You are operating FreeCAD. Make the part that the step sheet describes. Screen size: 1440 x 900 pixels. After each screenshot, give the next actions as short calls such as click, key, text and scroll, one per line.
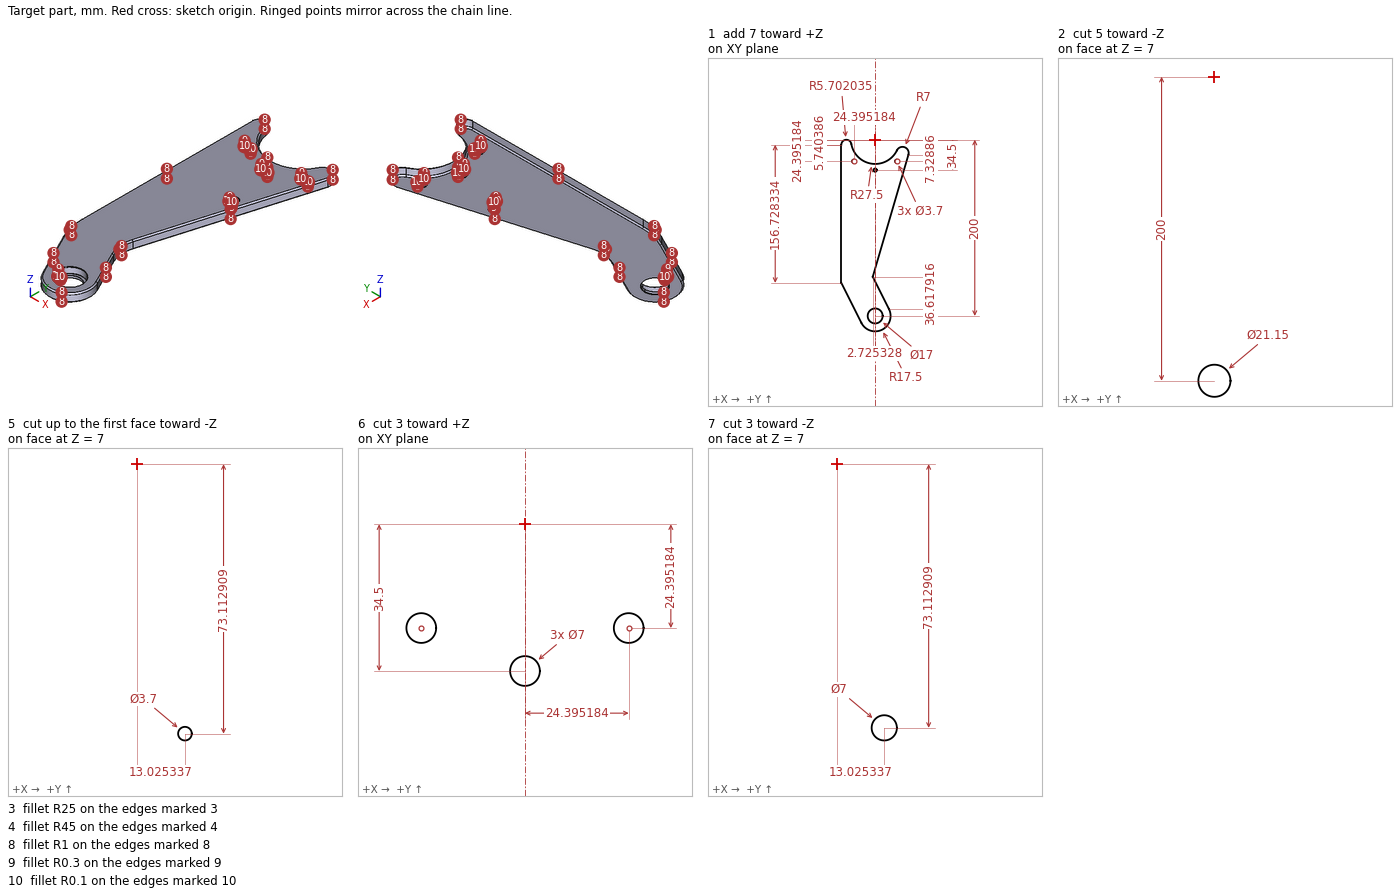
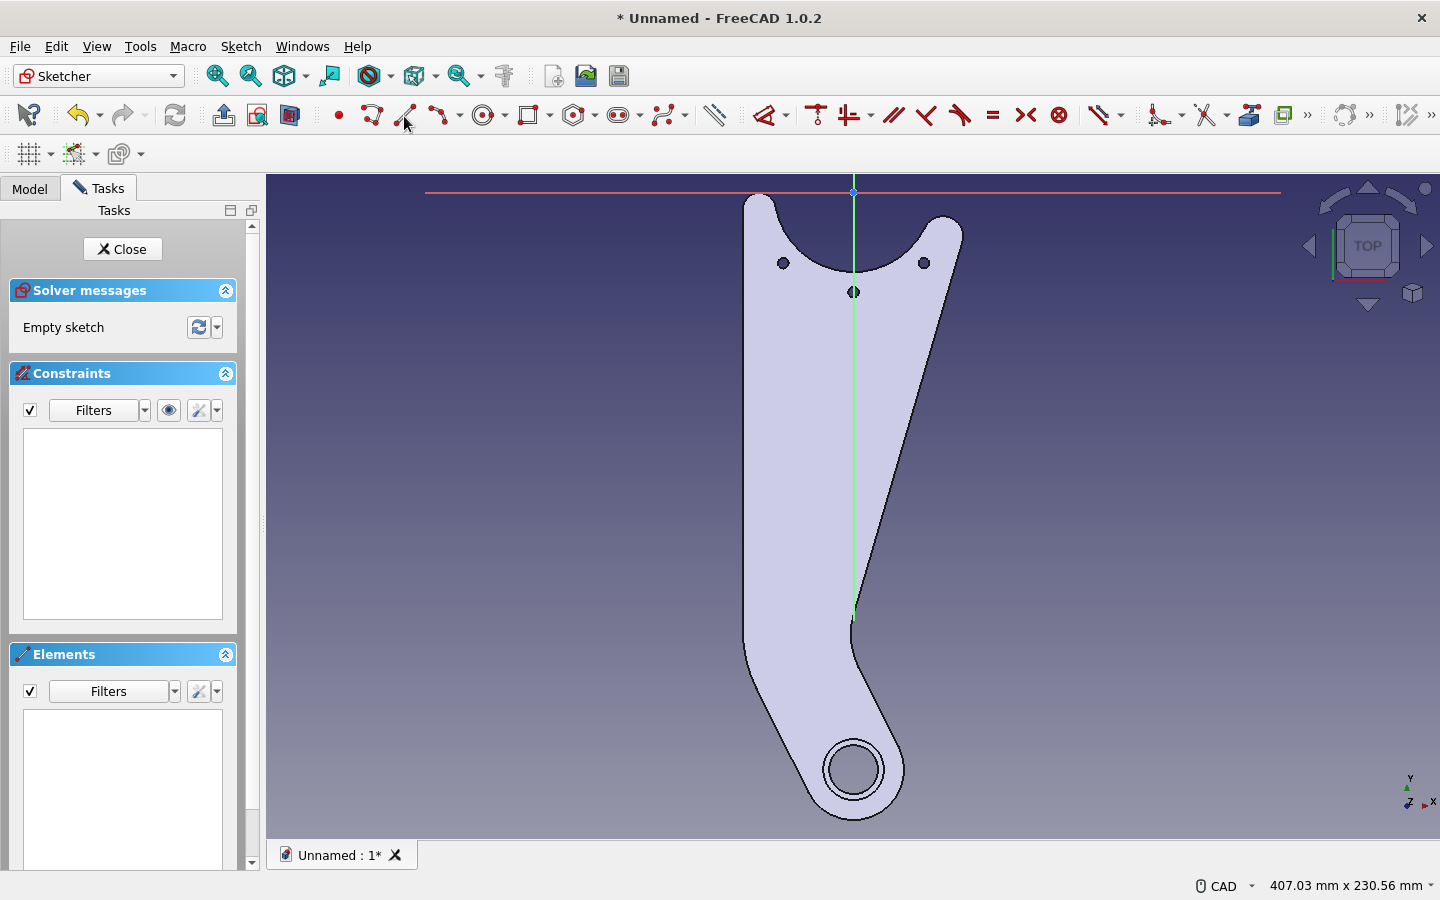
scroll(897, 398, up, 15)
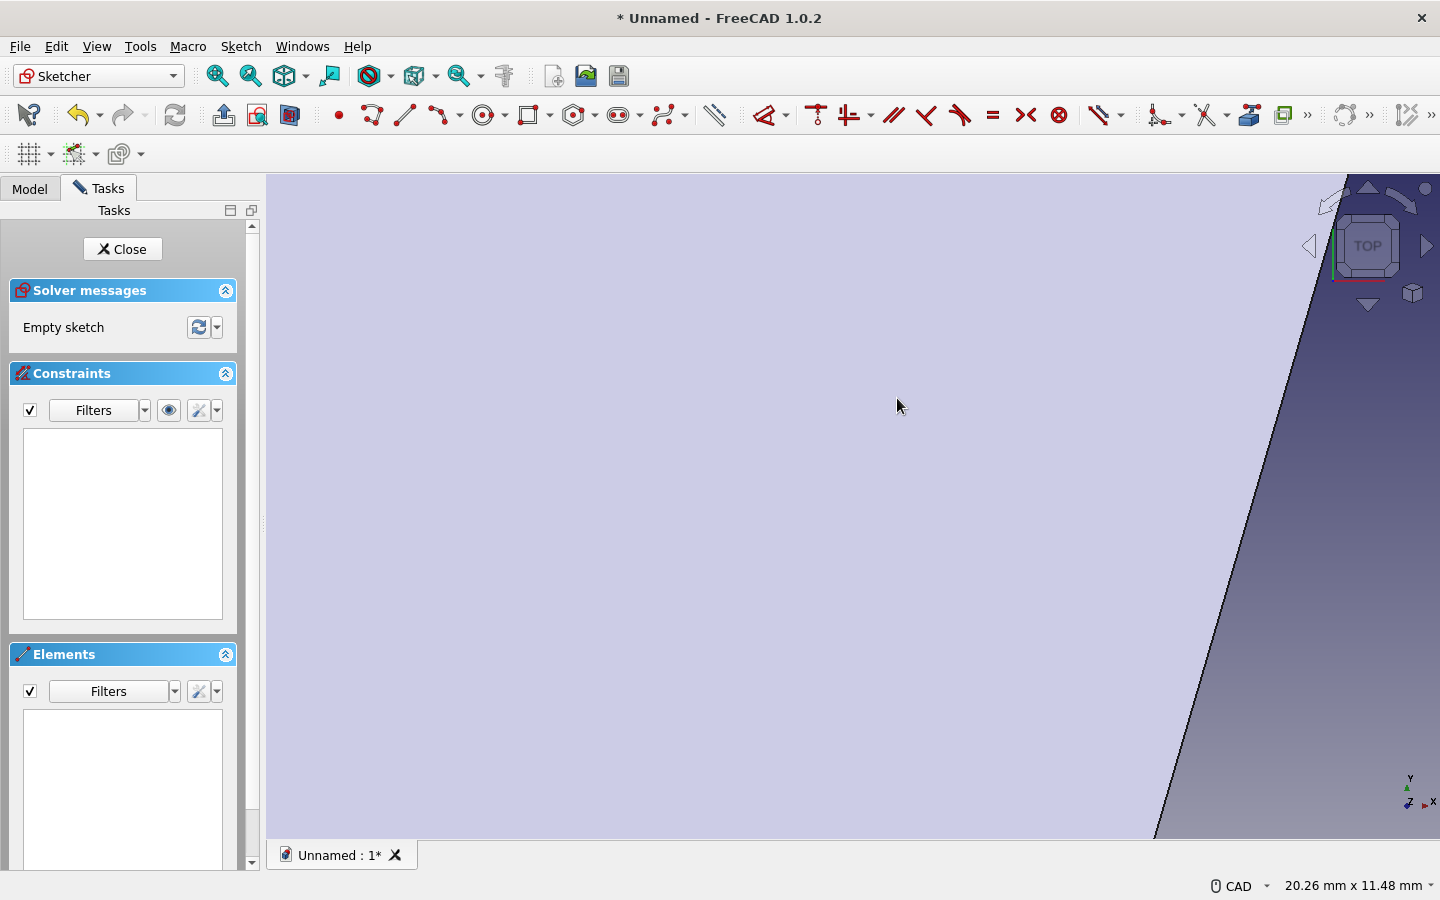
scroll(750, 504, up, 3)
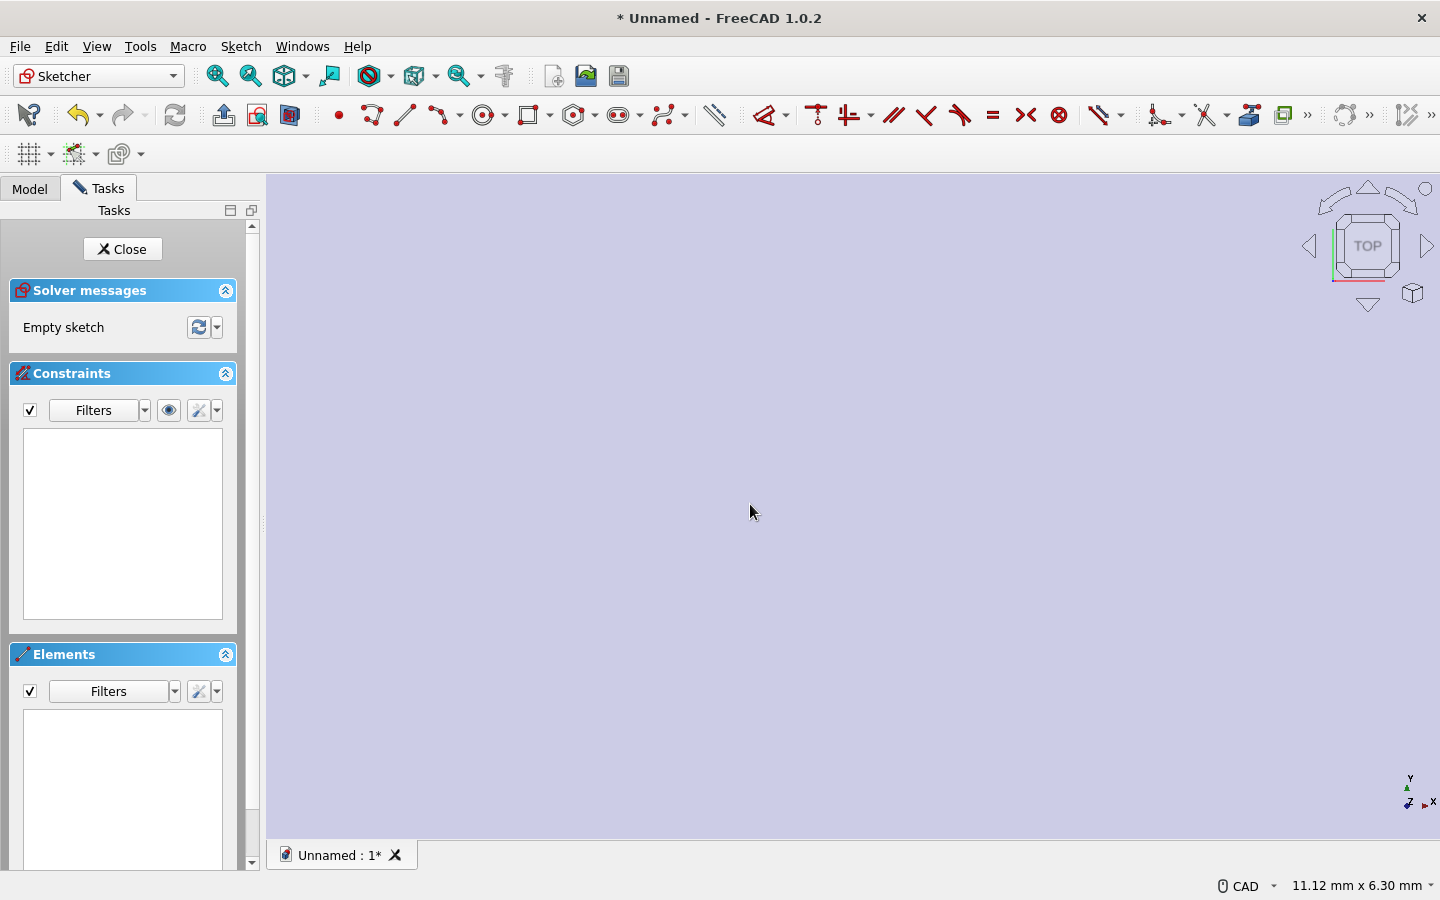
click(482, 116)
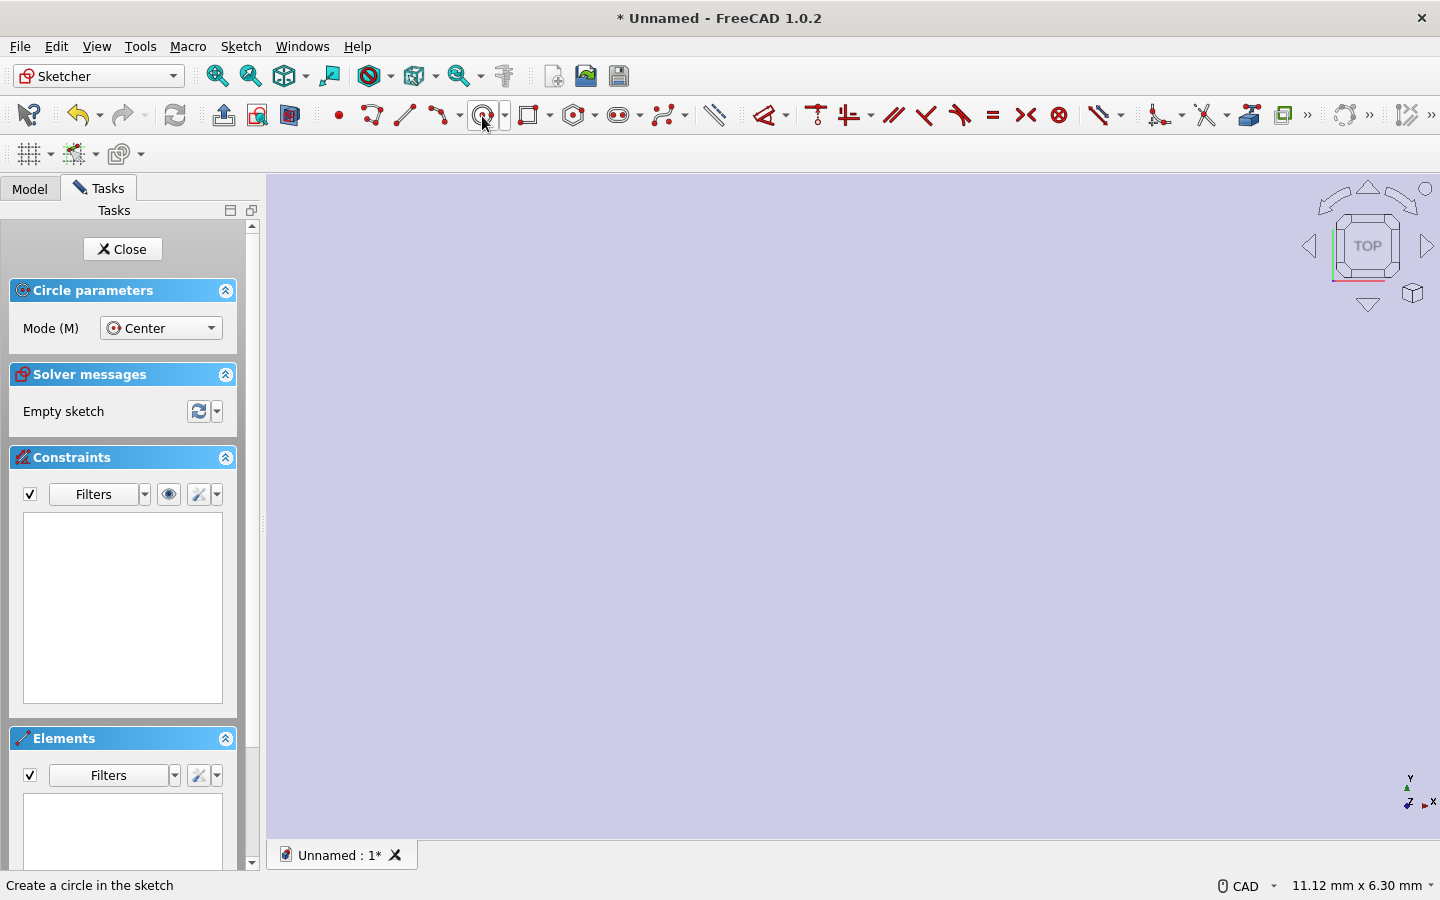
click(784, 506)
click(922, 368)
key(Escape)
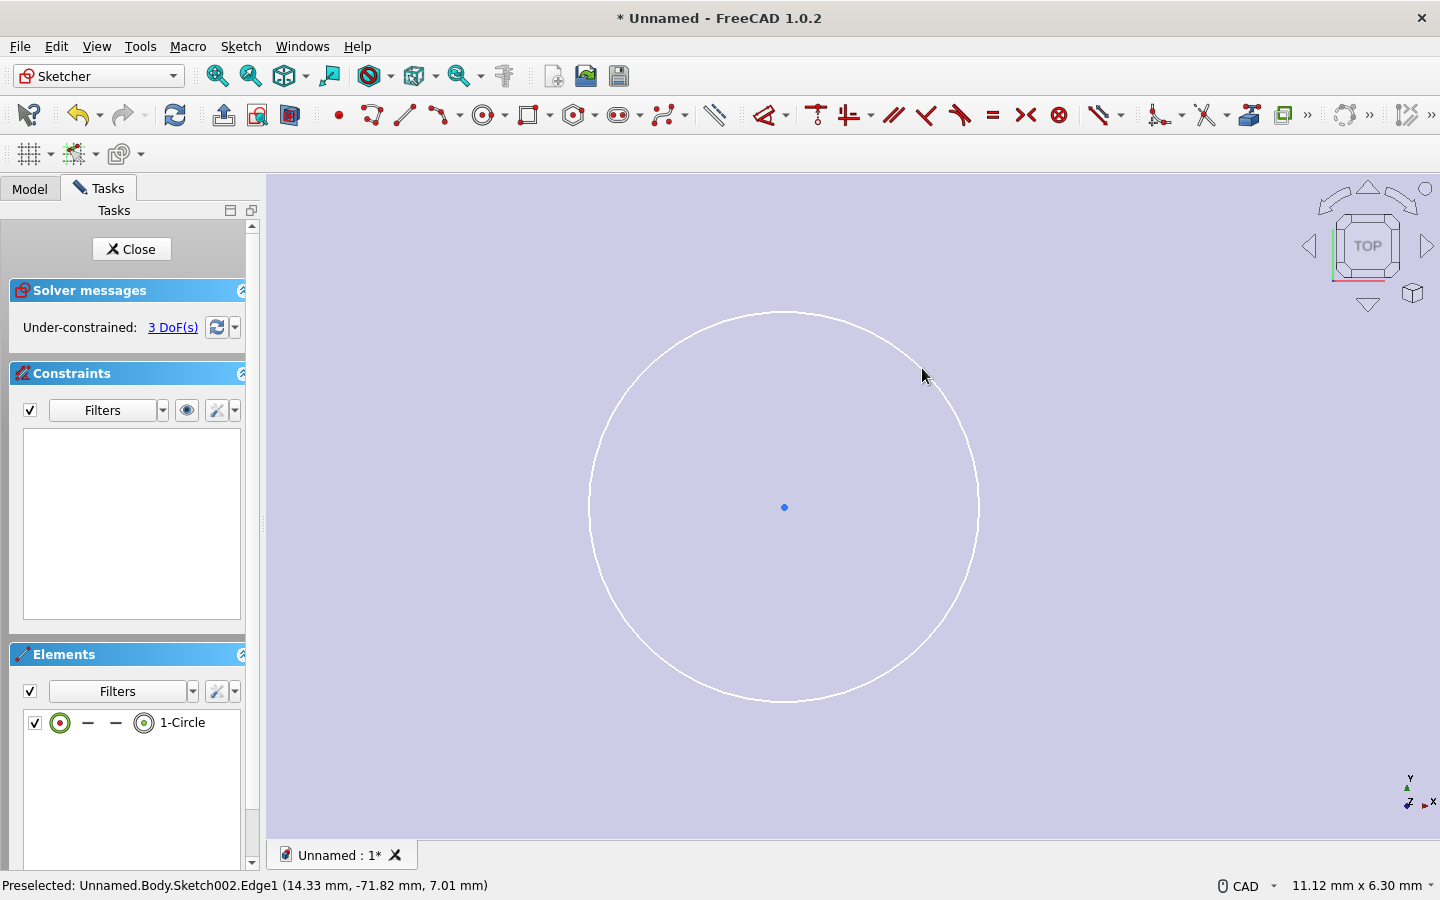
key(d)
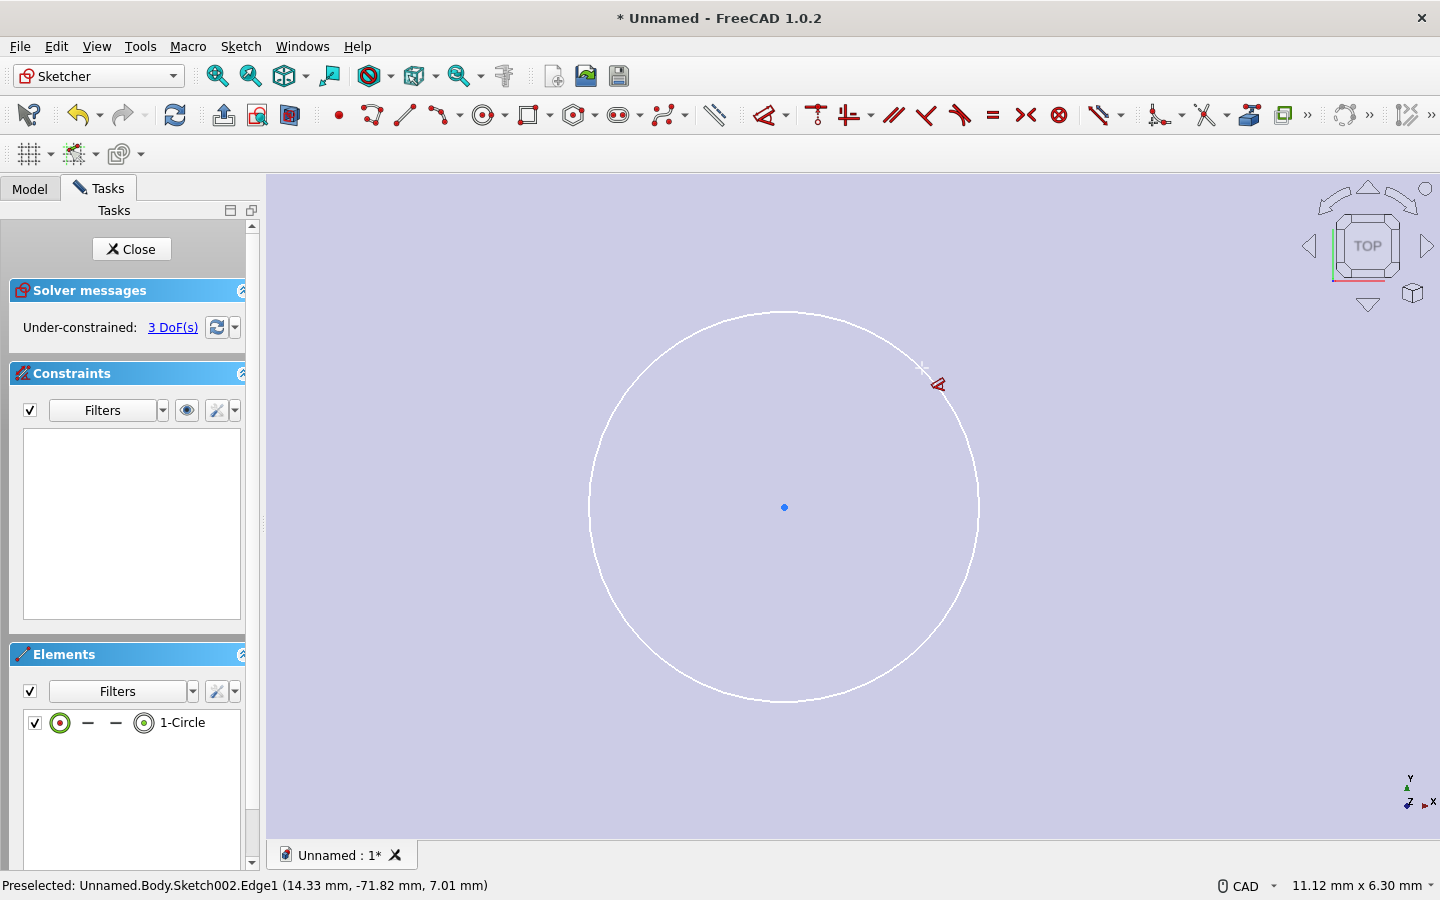
click(922, 369)
click(945, 346)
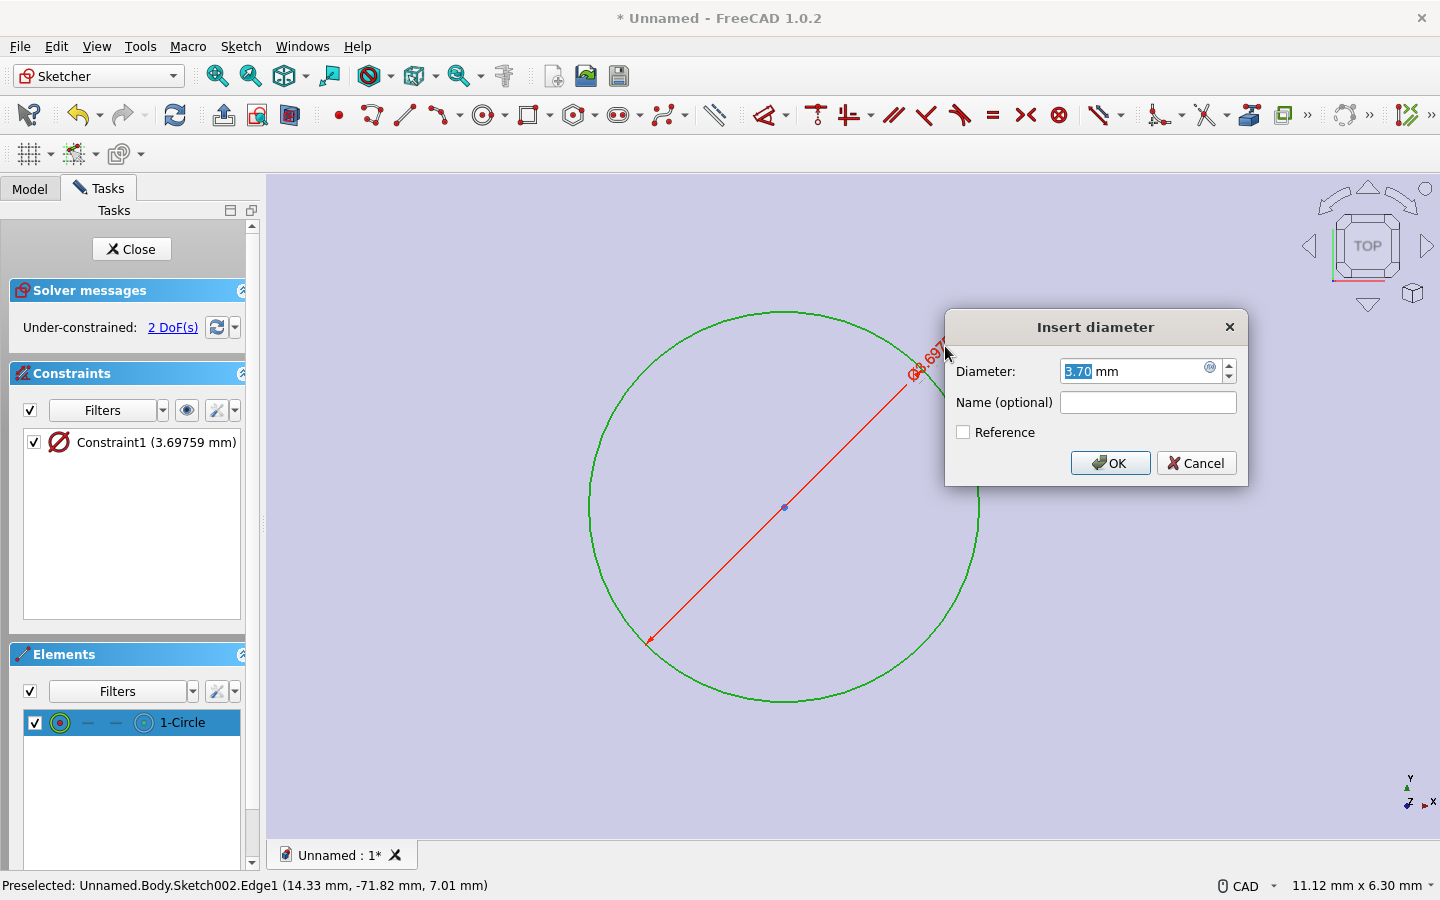
text(3.7)
key(Return)